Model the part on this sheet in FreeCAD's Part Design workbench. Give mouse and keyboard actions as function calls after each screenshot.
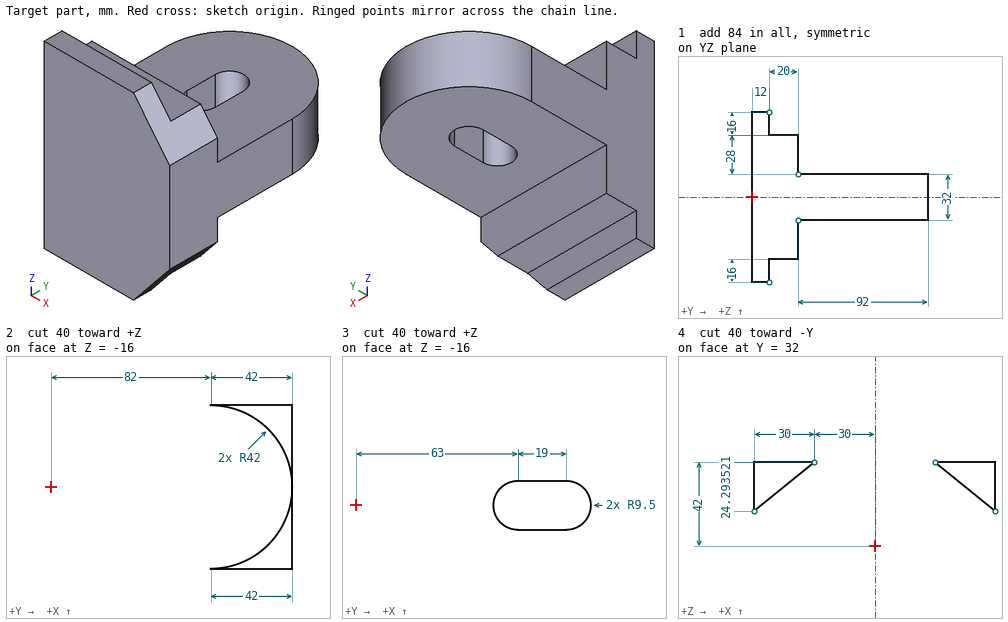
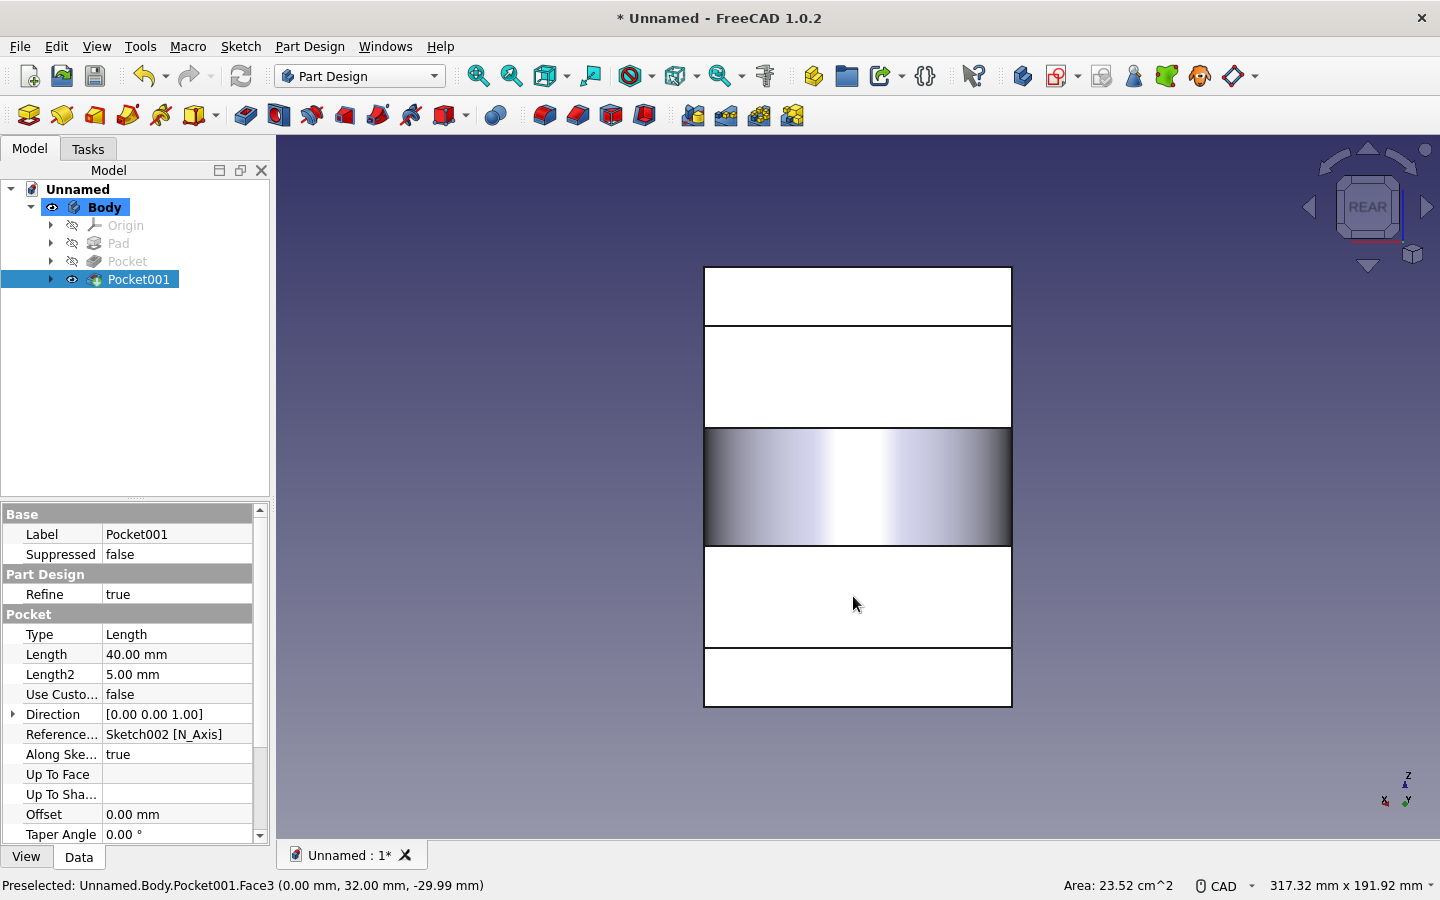
click(1056, 76)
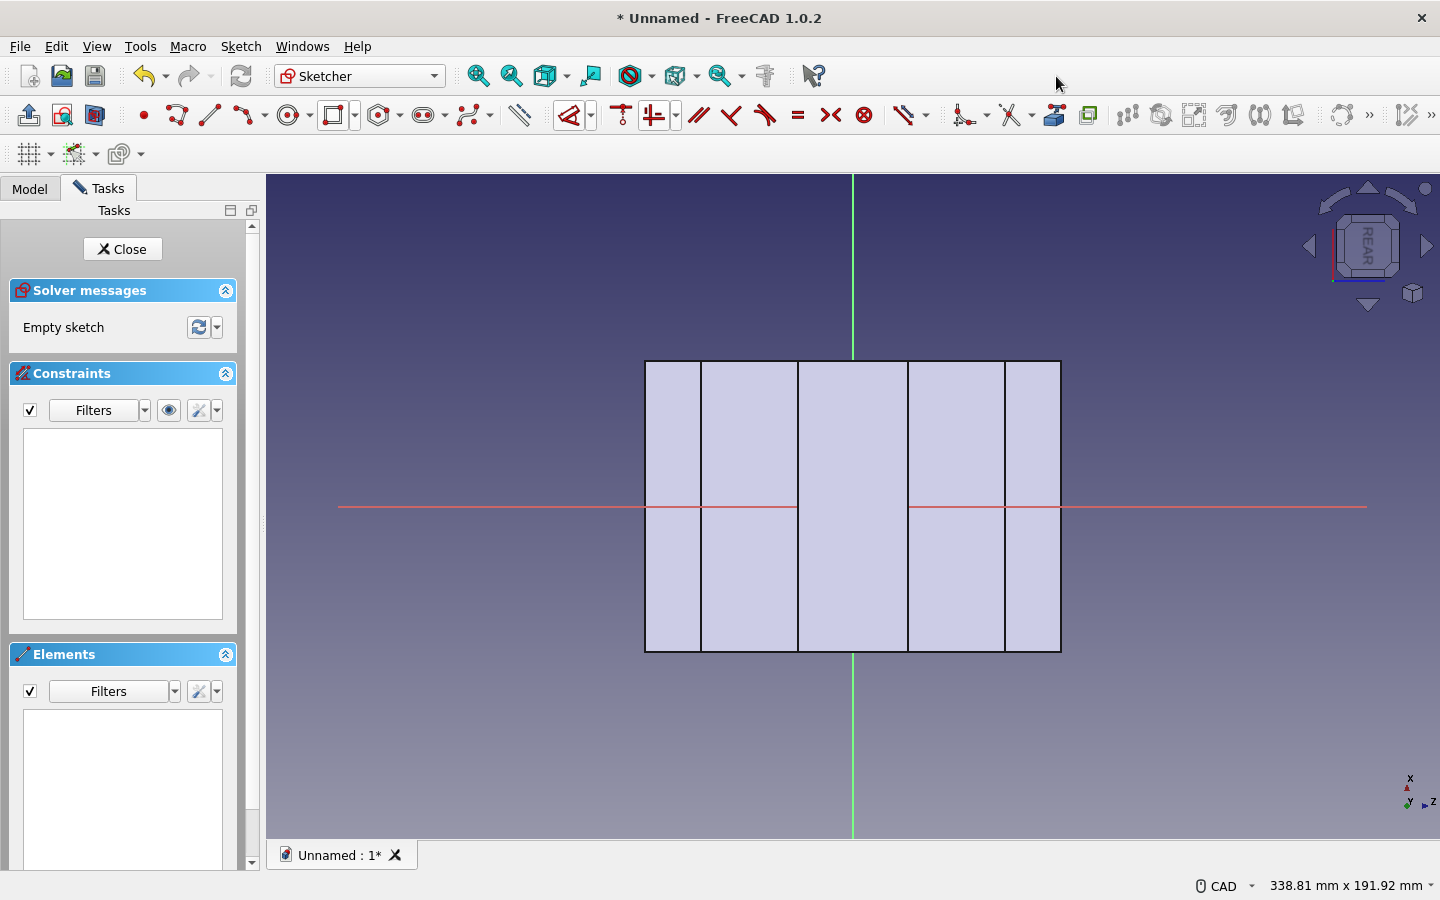
key(q)
key(s)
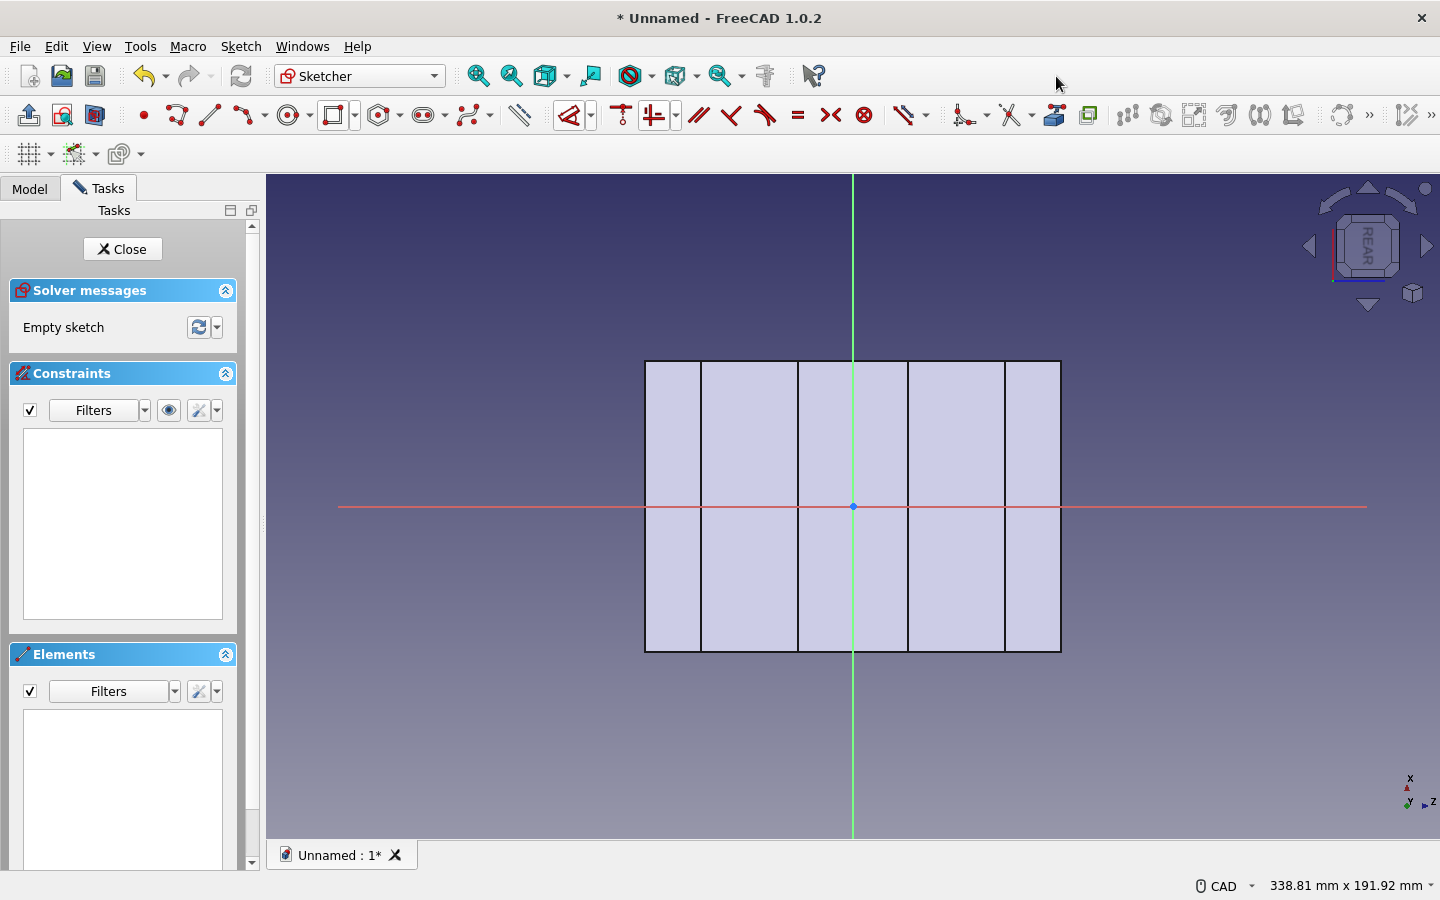
scroll(936, 345, up, 3)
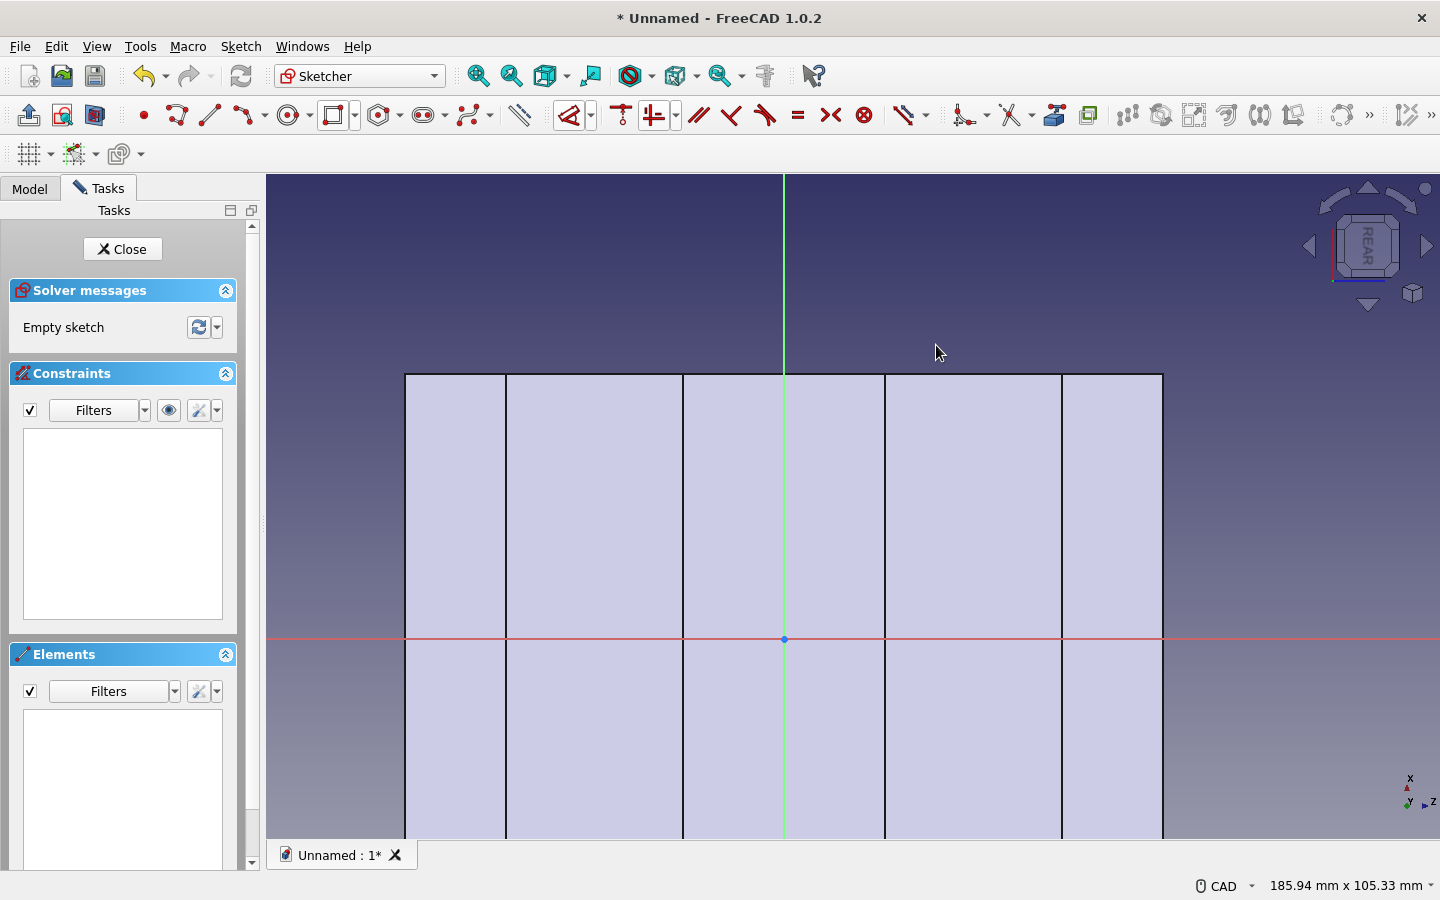
key(g)
key(m)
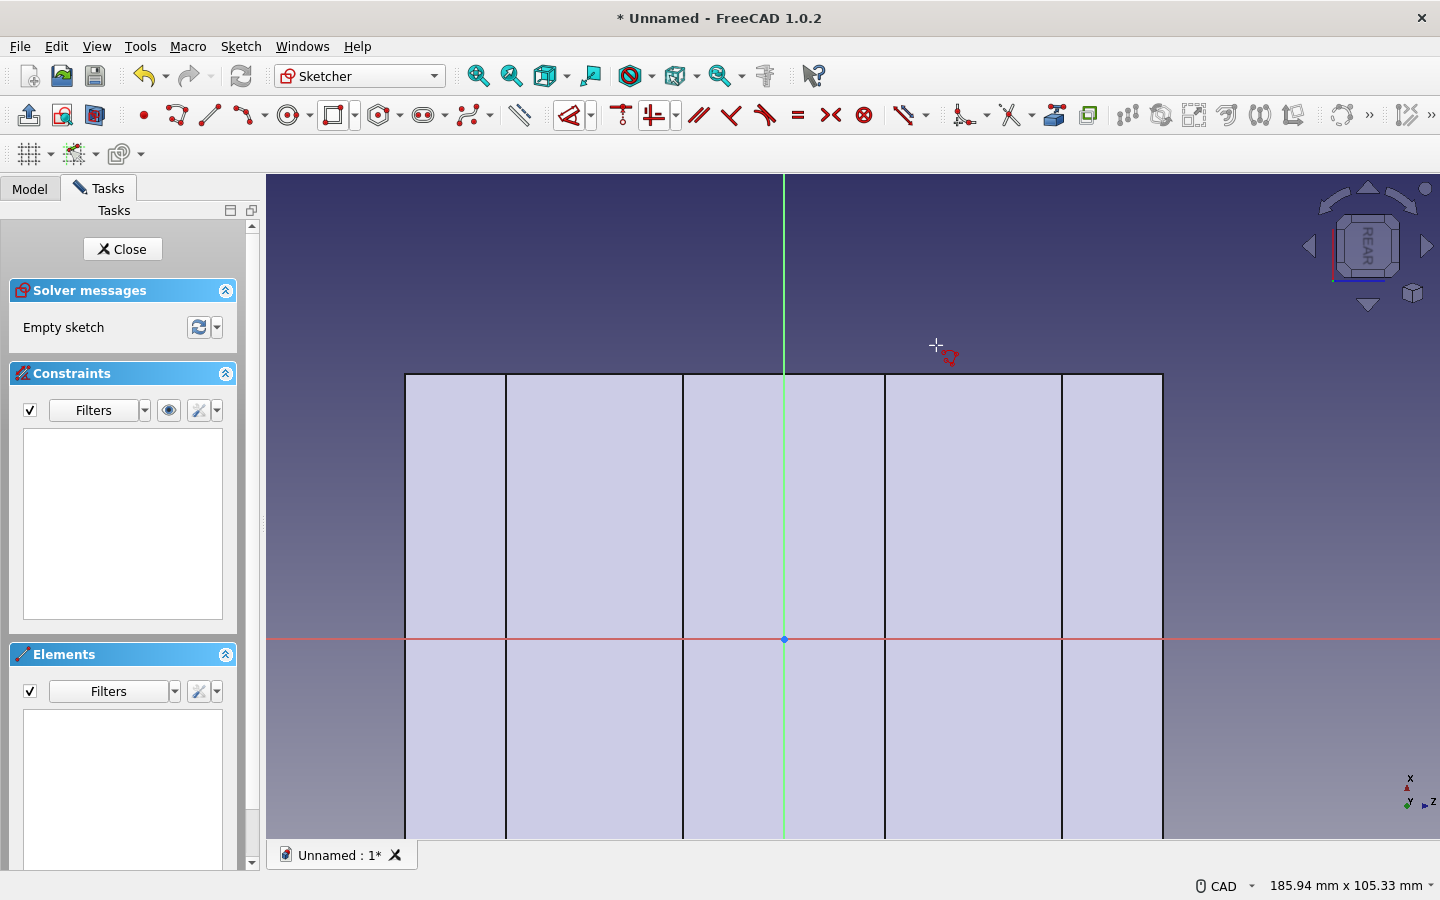
click(595, 374)
click(405, 374)
click(405, 527)
click(595, 375)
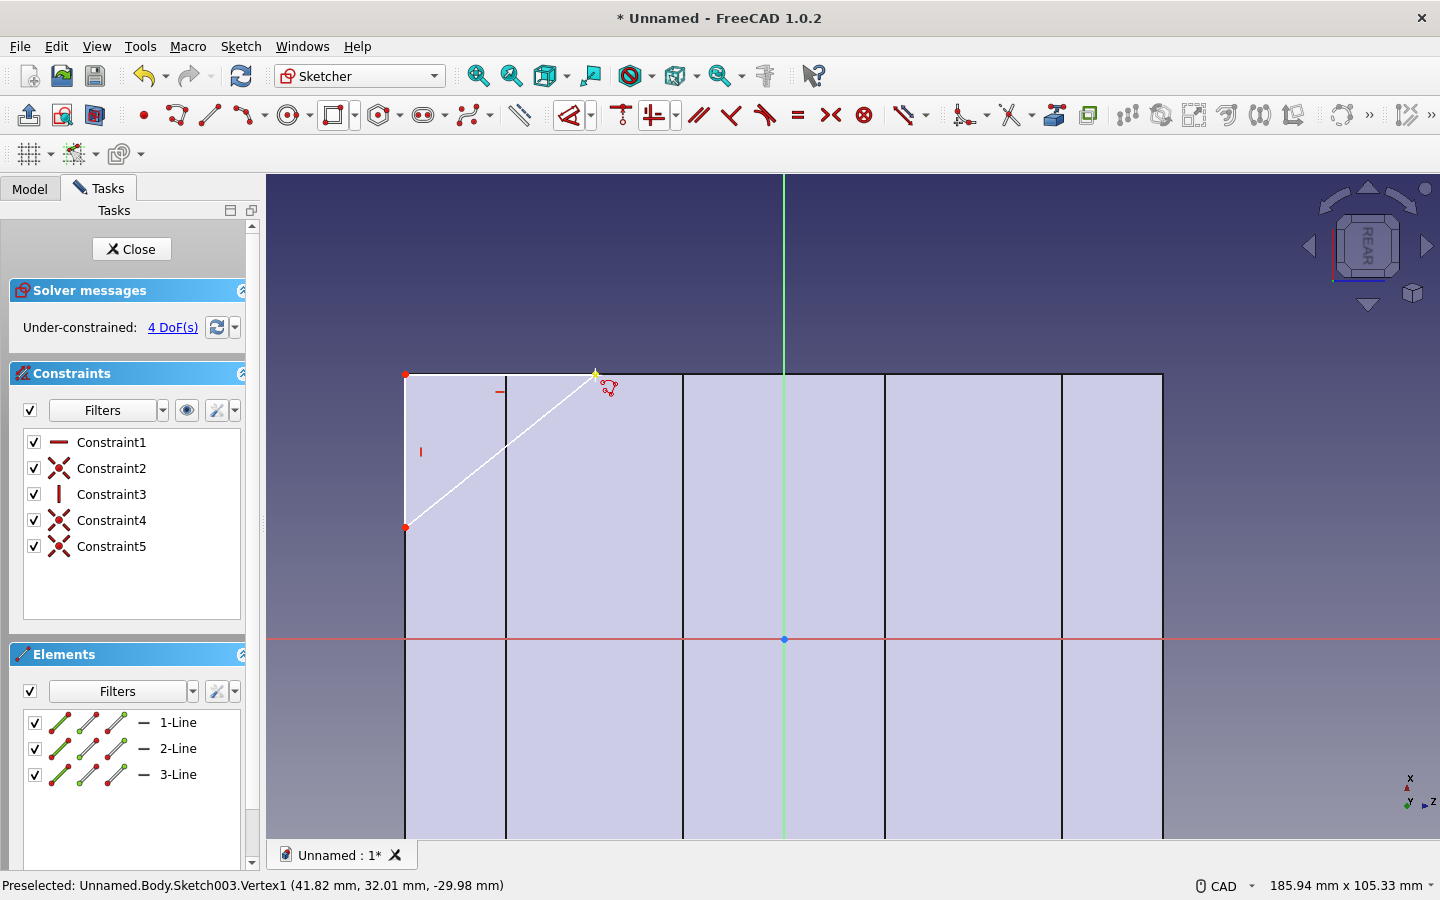
click(974, 374)
click(1163, 527)
click(1163, 374)
click(974, 375)
key(Escape)
key(Escape)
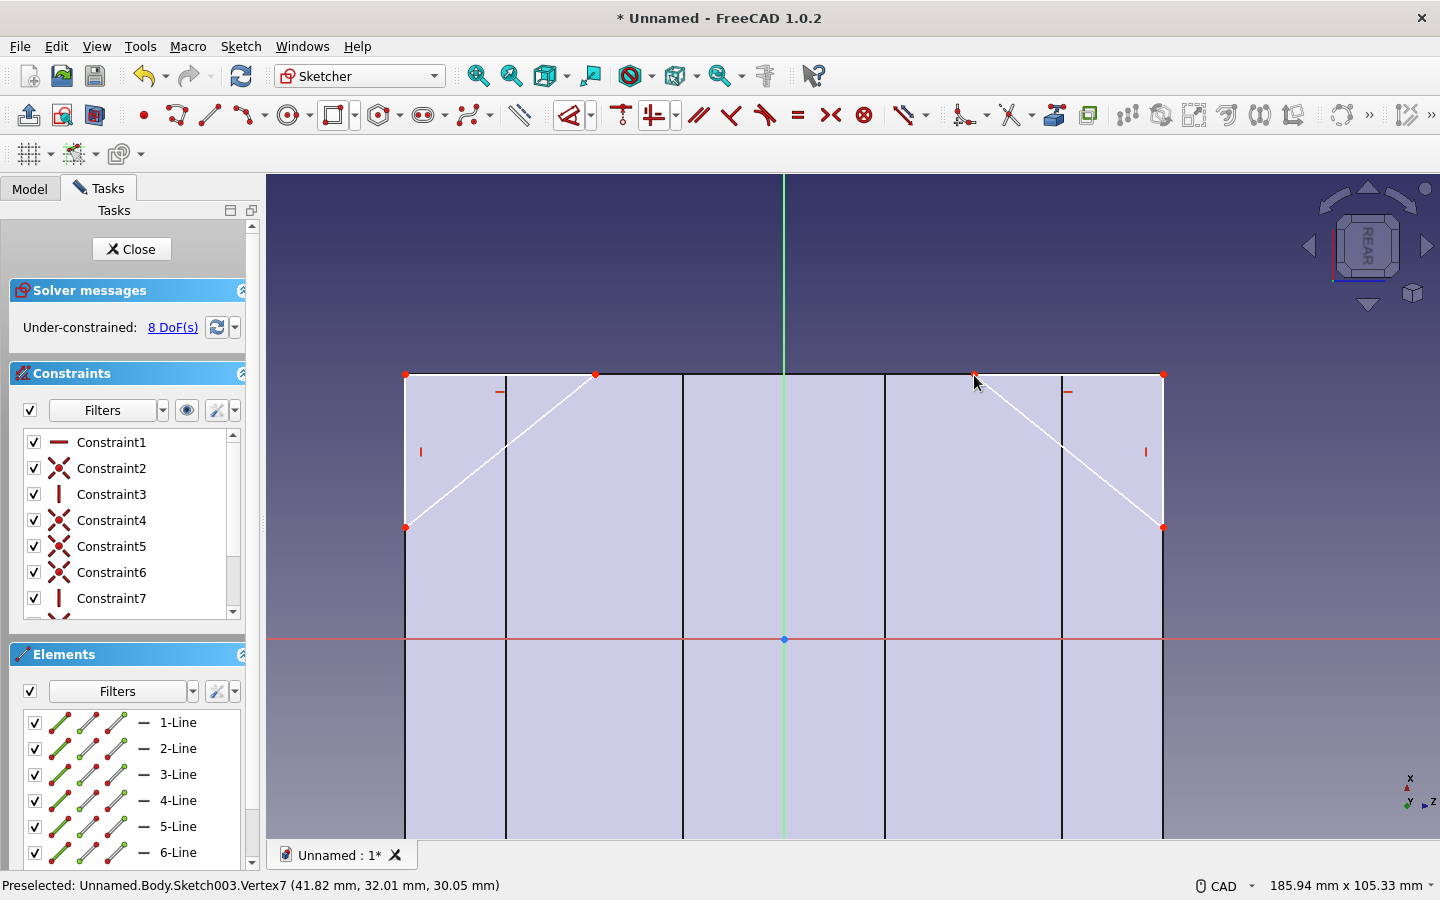
click(595, 375)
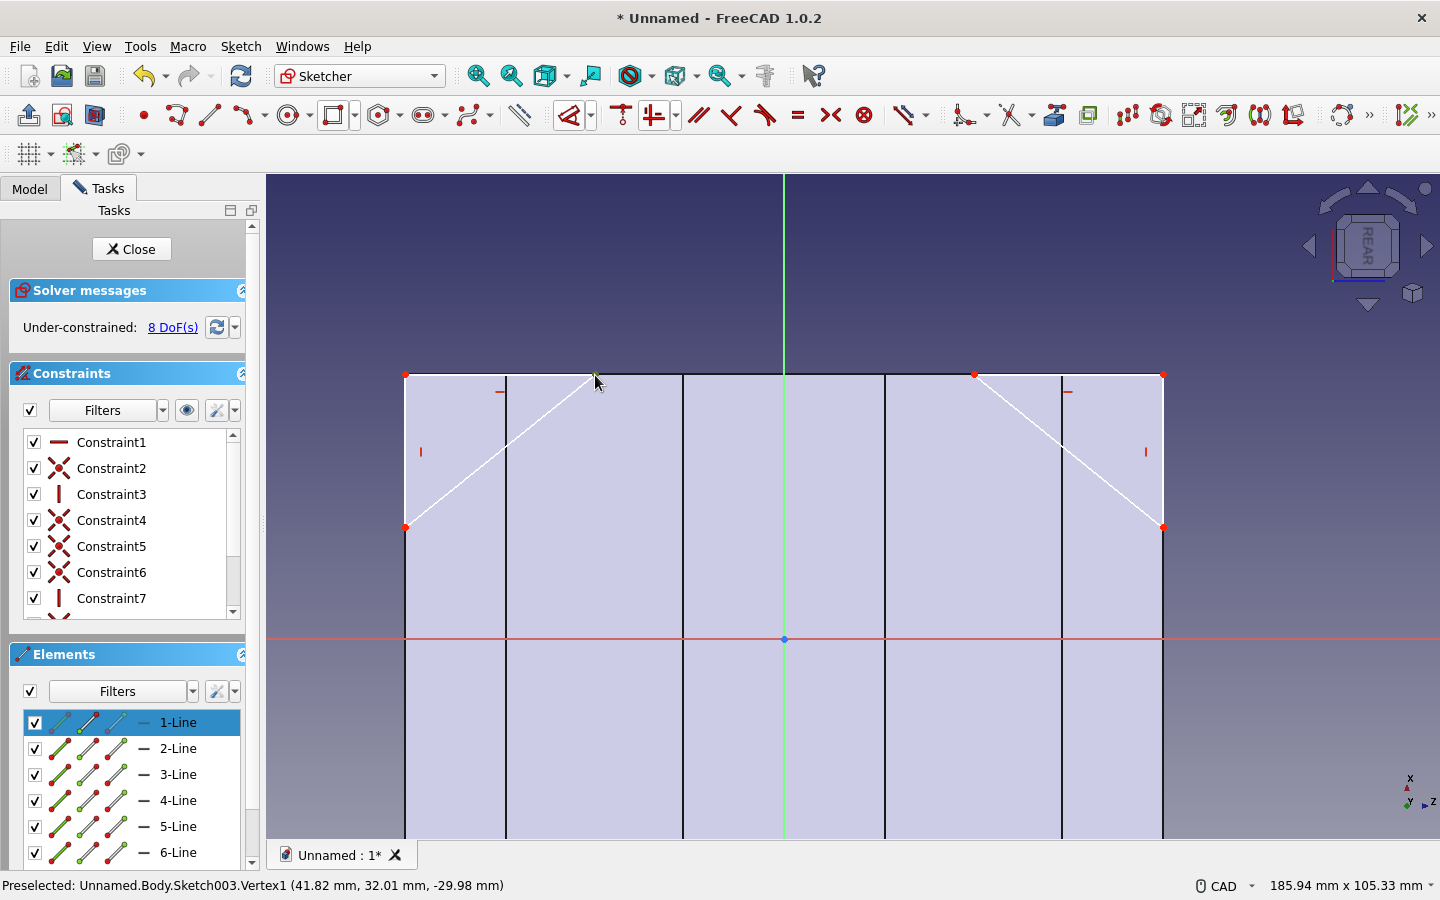
click(974, 375)